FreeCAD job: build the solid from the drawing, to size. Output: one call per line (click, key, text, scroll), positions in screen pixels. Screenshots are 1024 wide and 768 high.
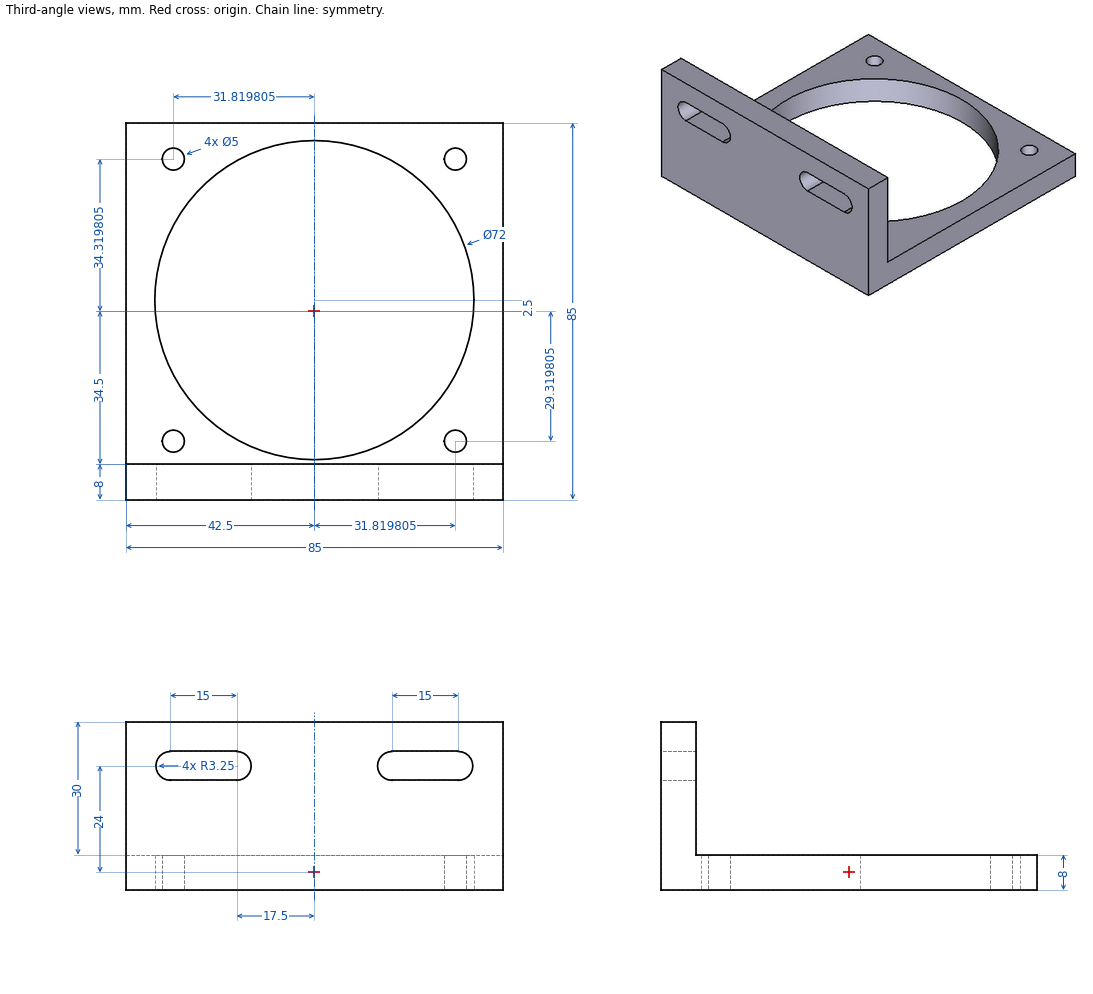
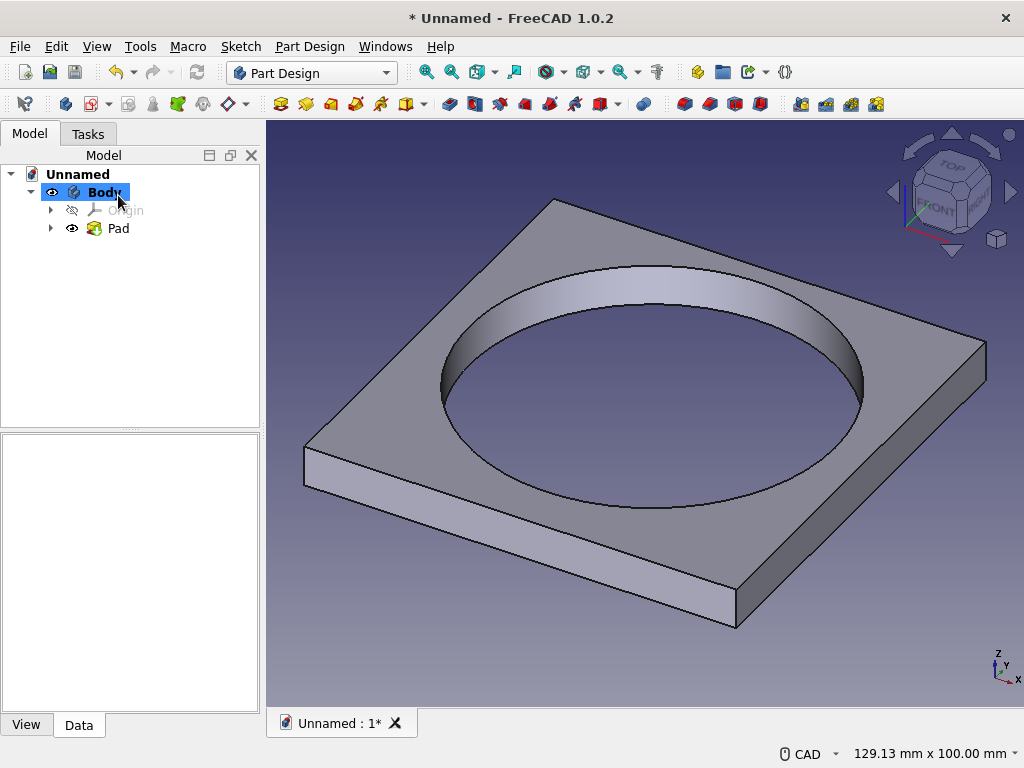
click(937, 348)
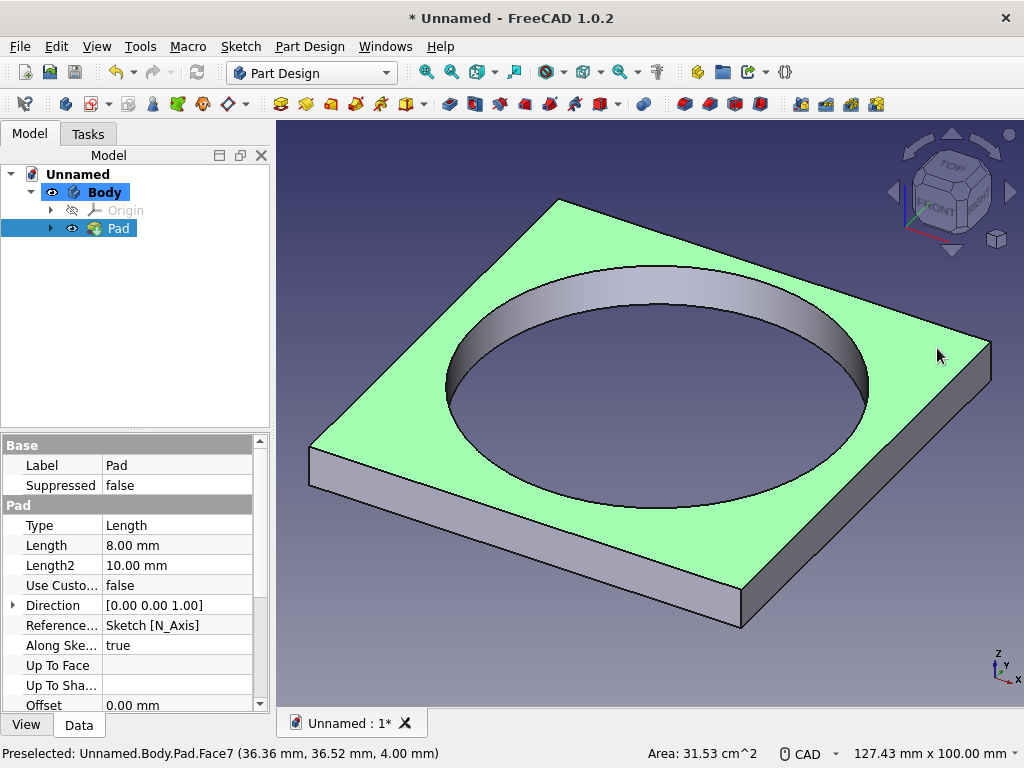
click(90, 104)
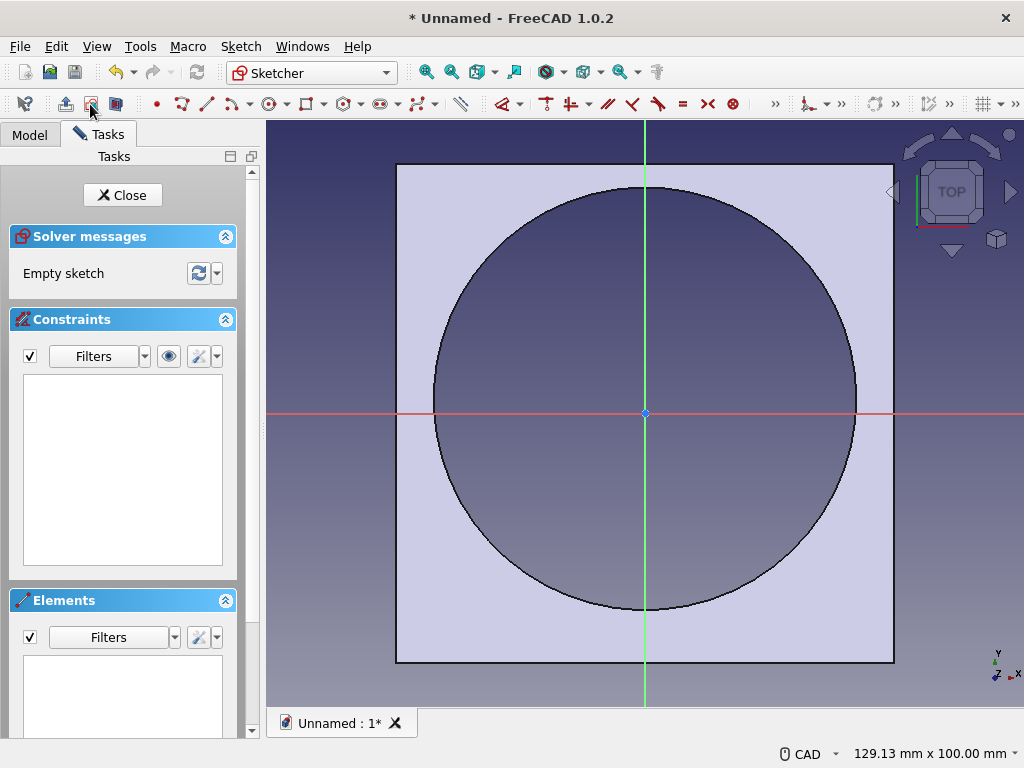
scroll(294, 480, down, 1)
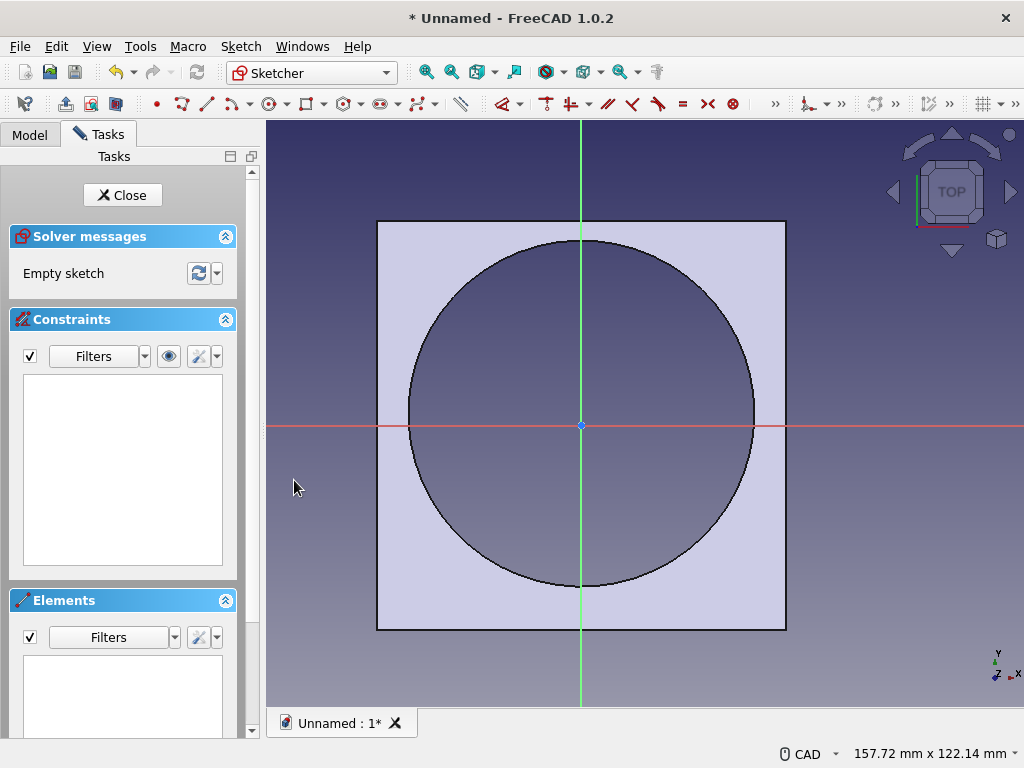
key(g)
key(c)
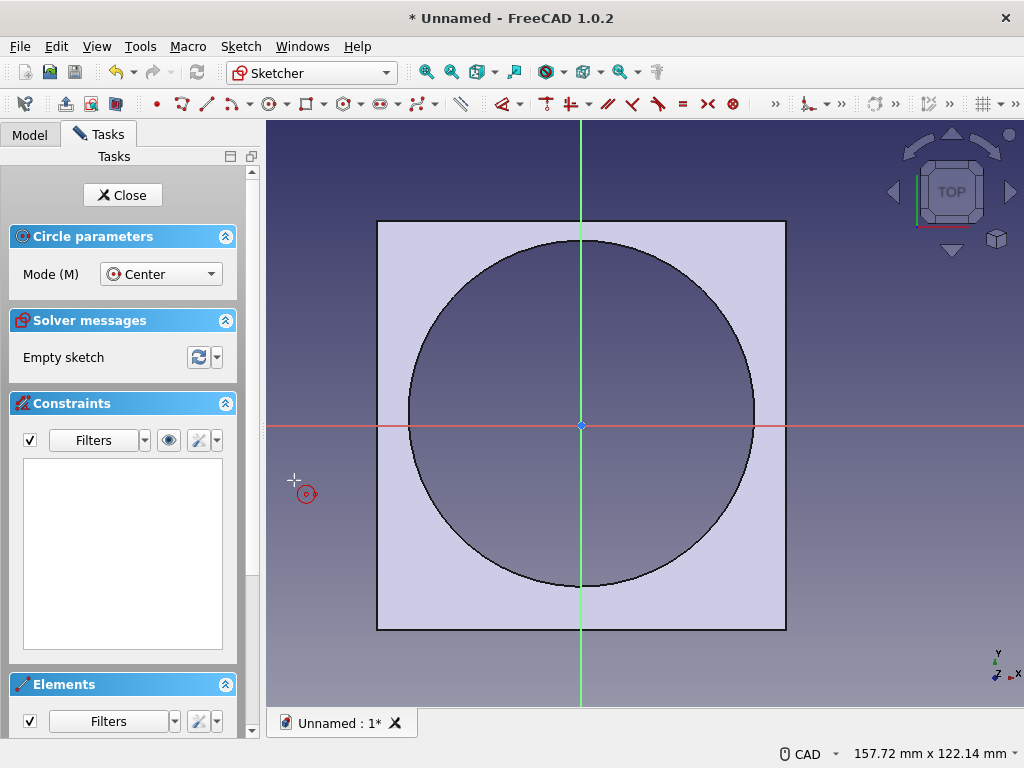
scroll(428, 261, up, 4)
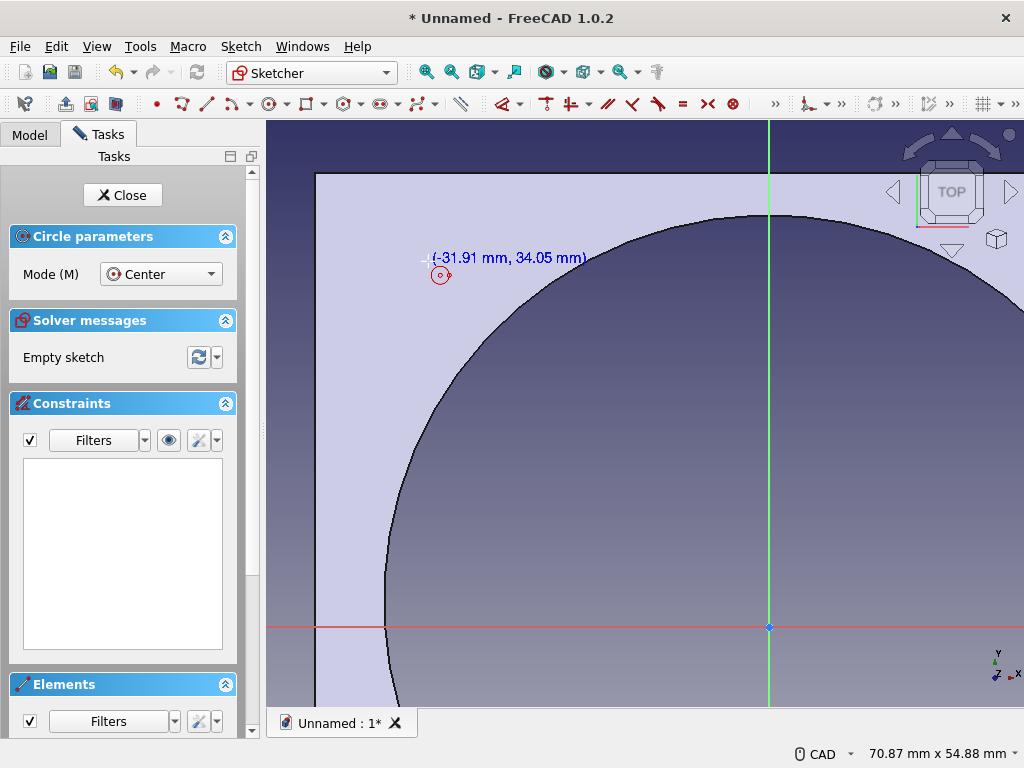
click(429, 260)
click(448, 241)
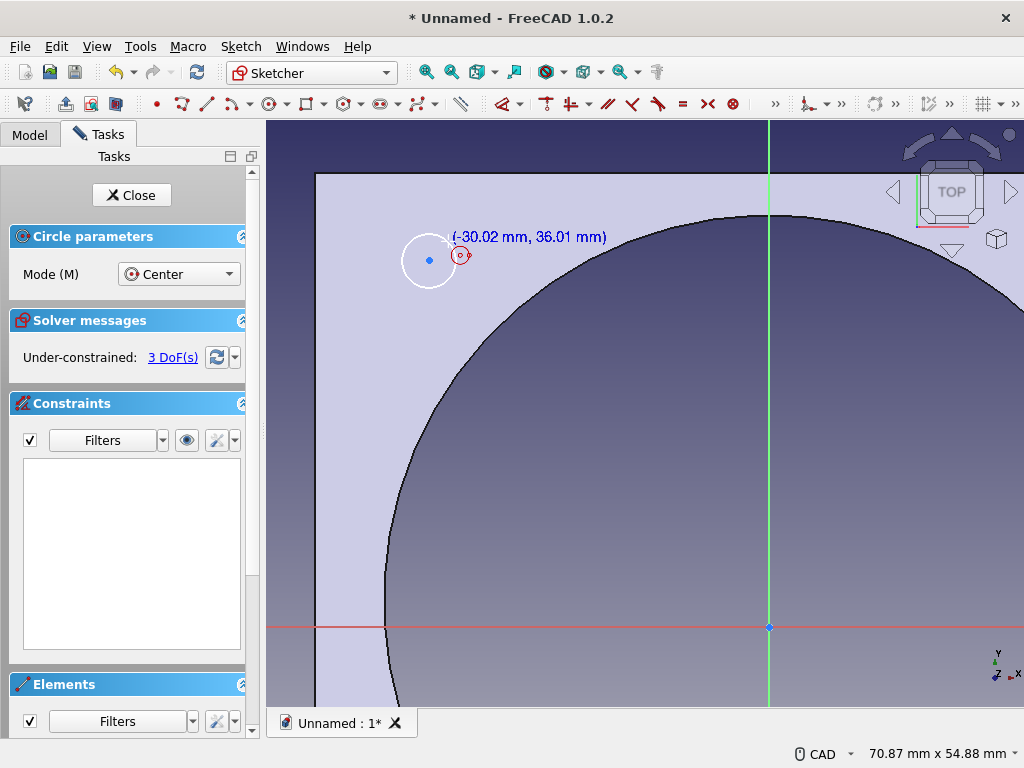
scroll(342, 186, down, 3)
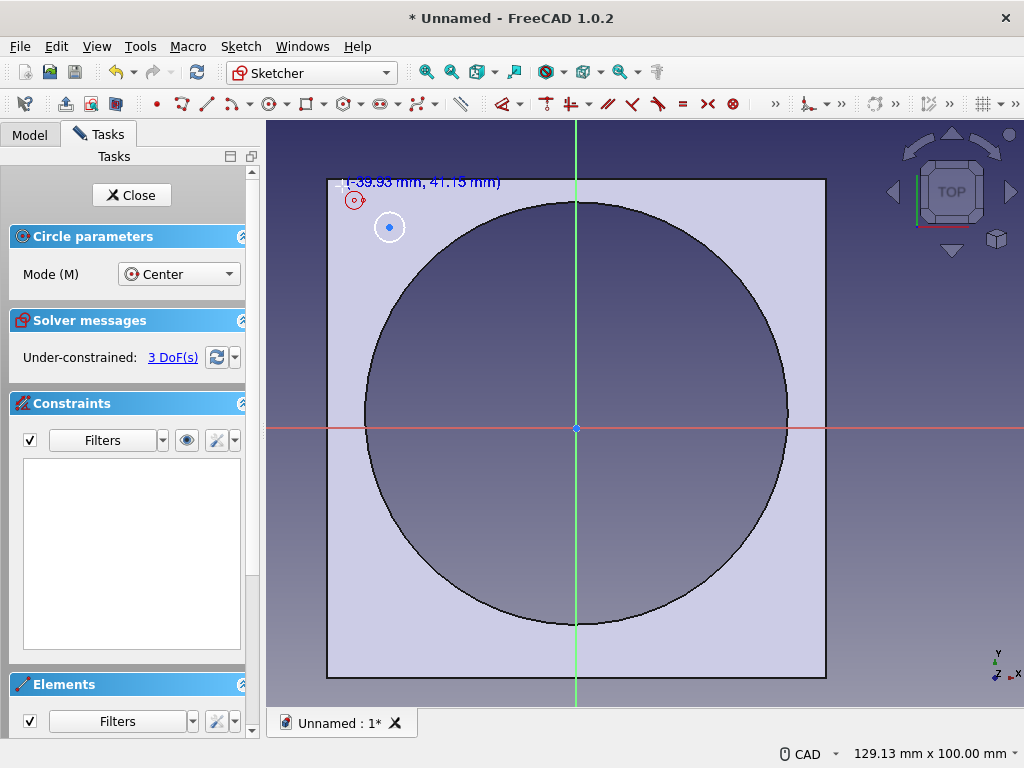
scroll(763, 600, up, 3)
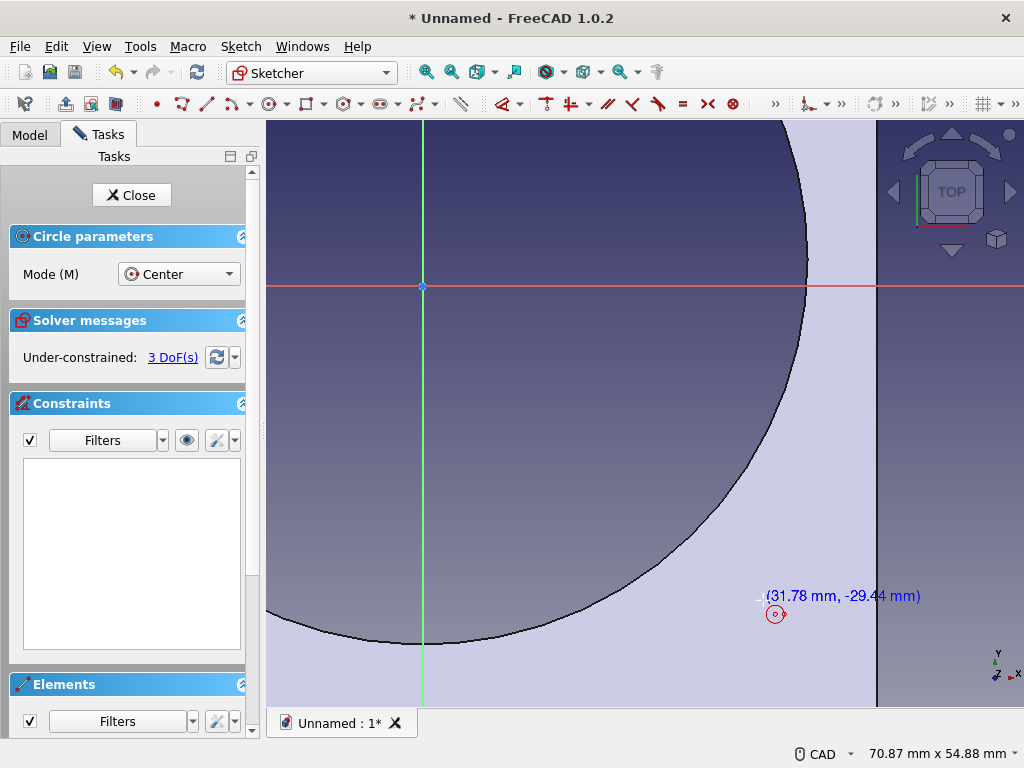
click(763, 600)
click(782, 581)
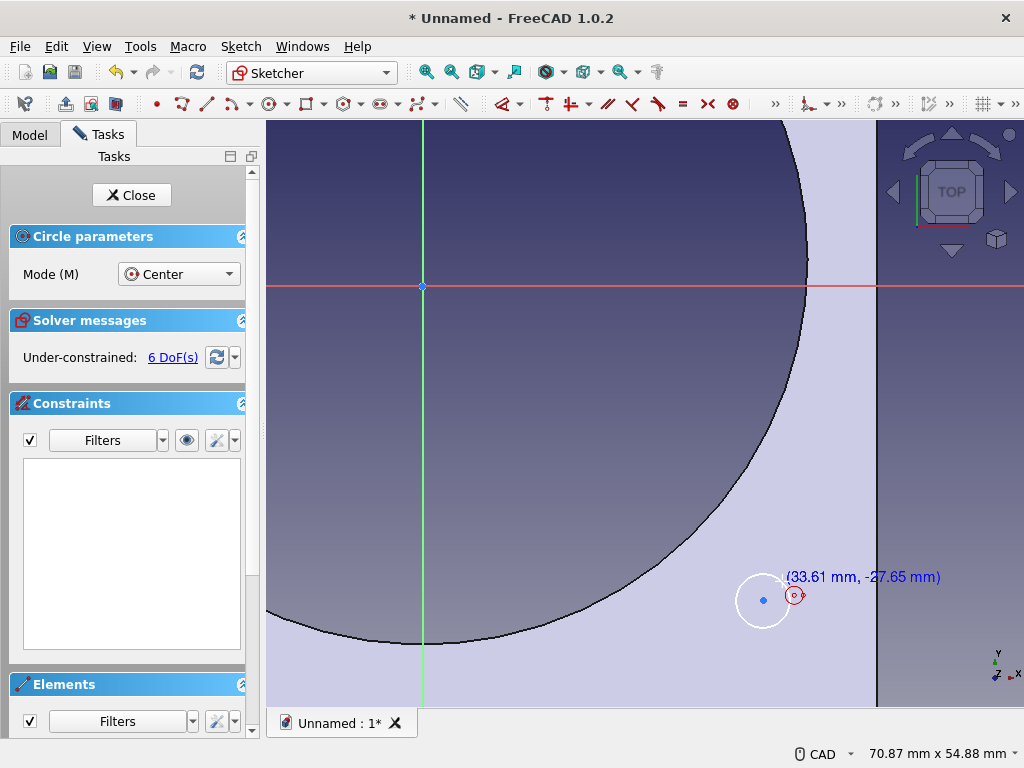
scroll(764, 601, down, 3)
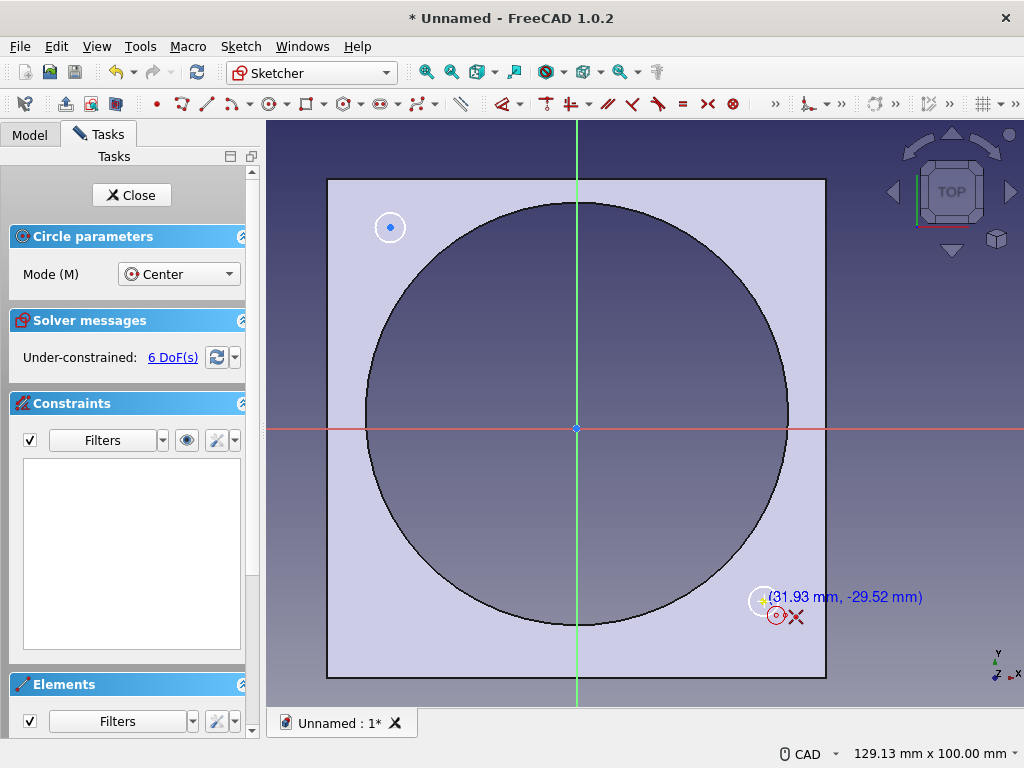
scroll(390, 601, up, 3)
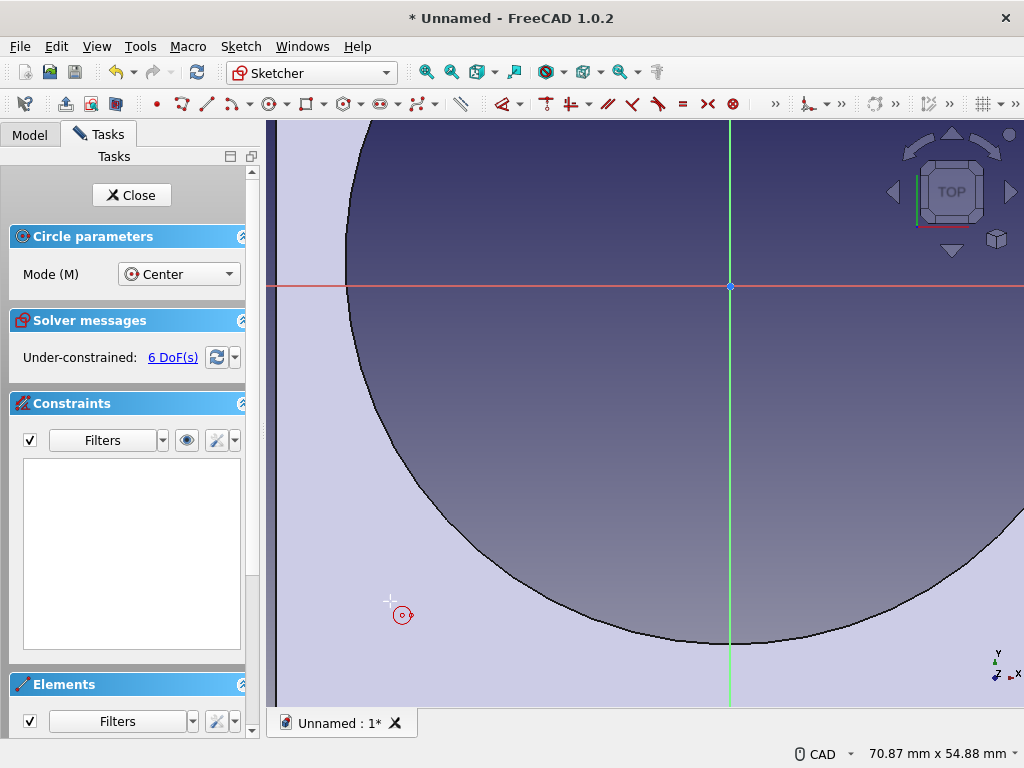
click(390, 600)
click(409, 581)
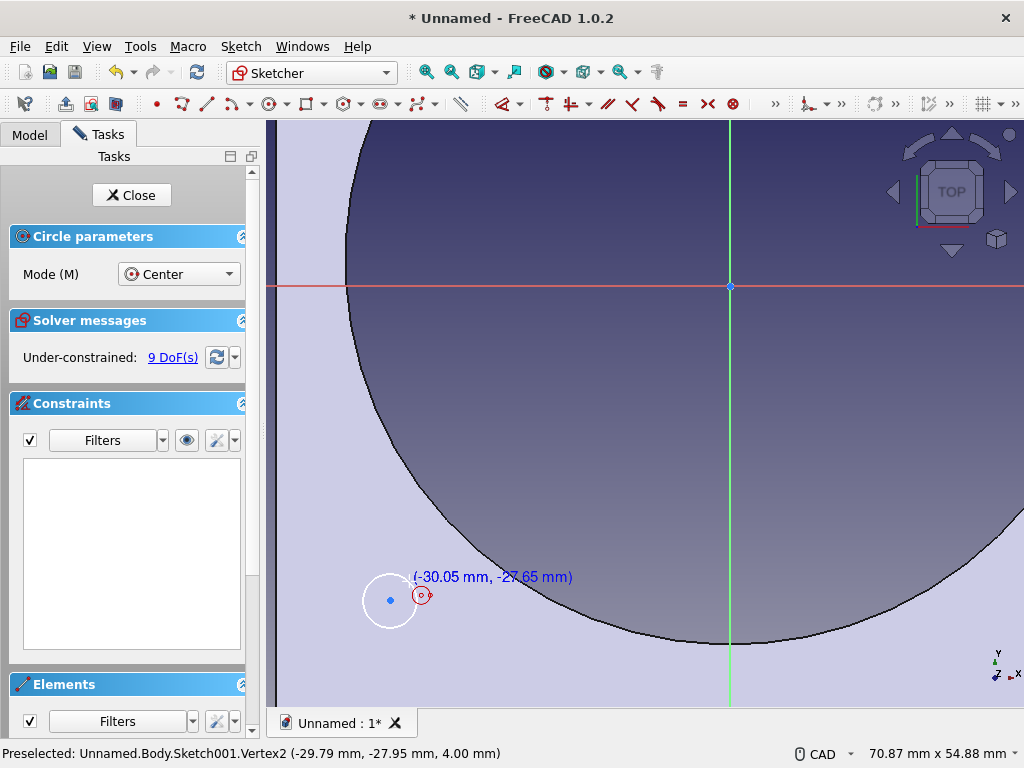
scroll(389, 601, down, 3)